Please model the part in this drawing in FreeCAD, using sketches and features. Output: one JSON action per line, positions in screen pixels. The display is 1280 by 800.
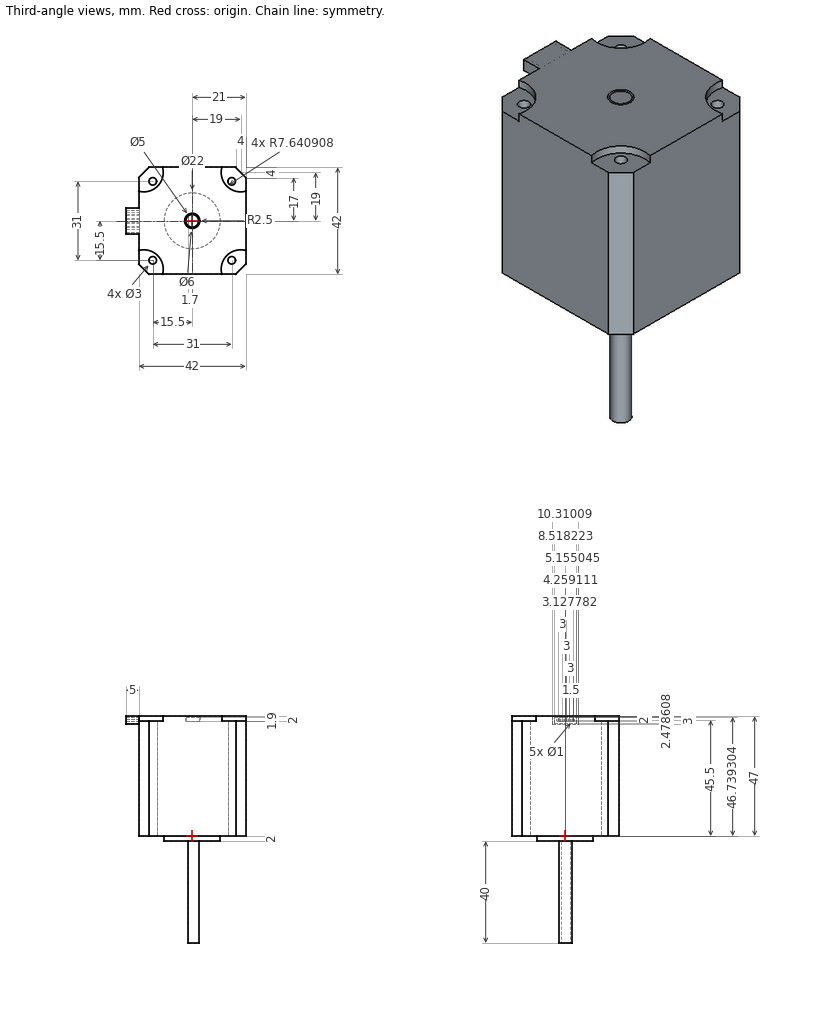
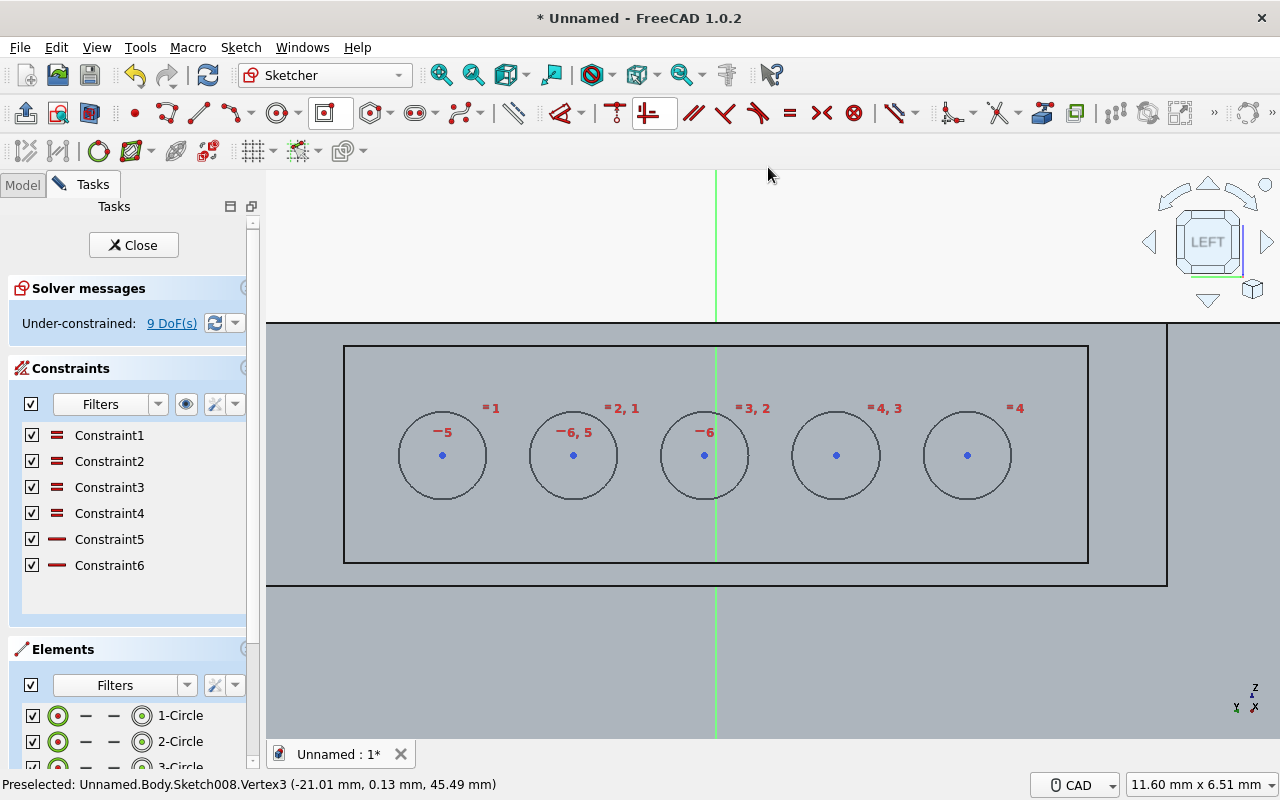
{"action": "left_click", "coordinate": [705, 456]}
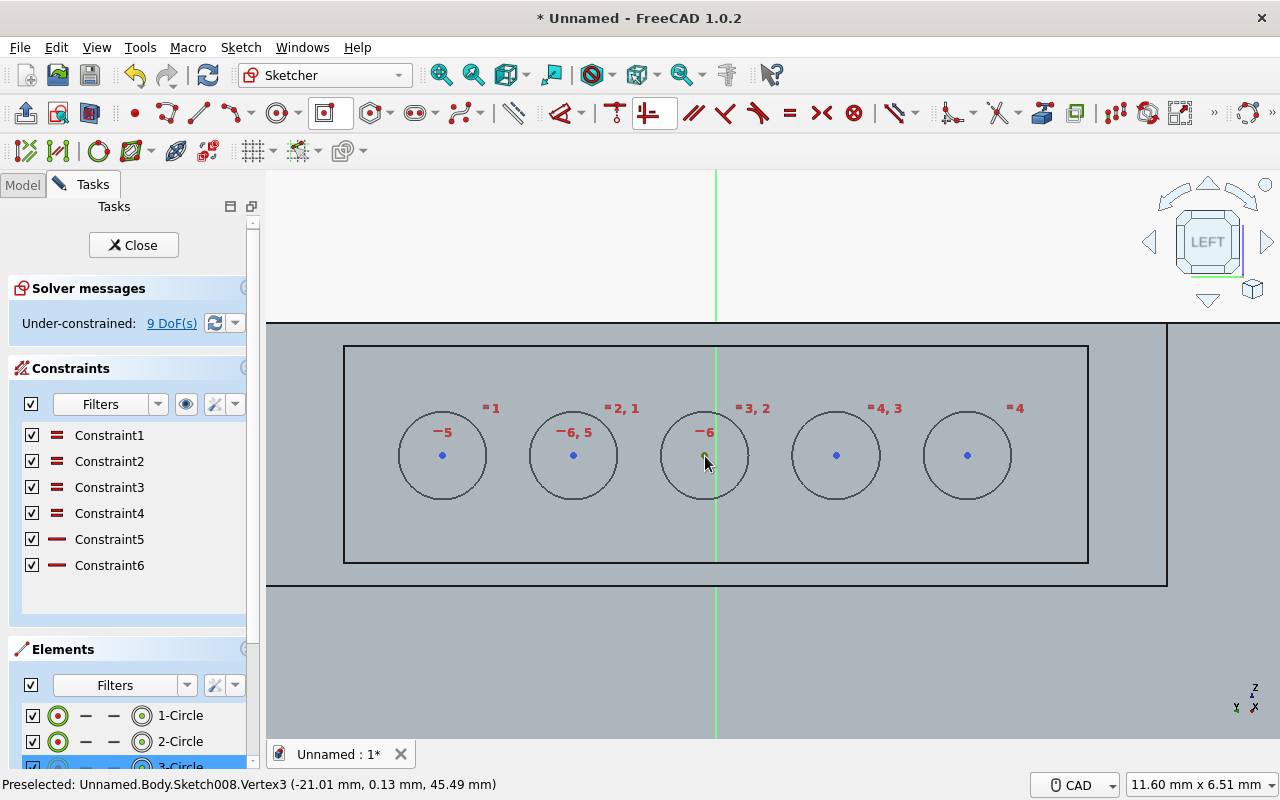
{"action": "left_click", "coordinate": [836, 455]}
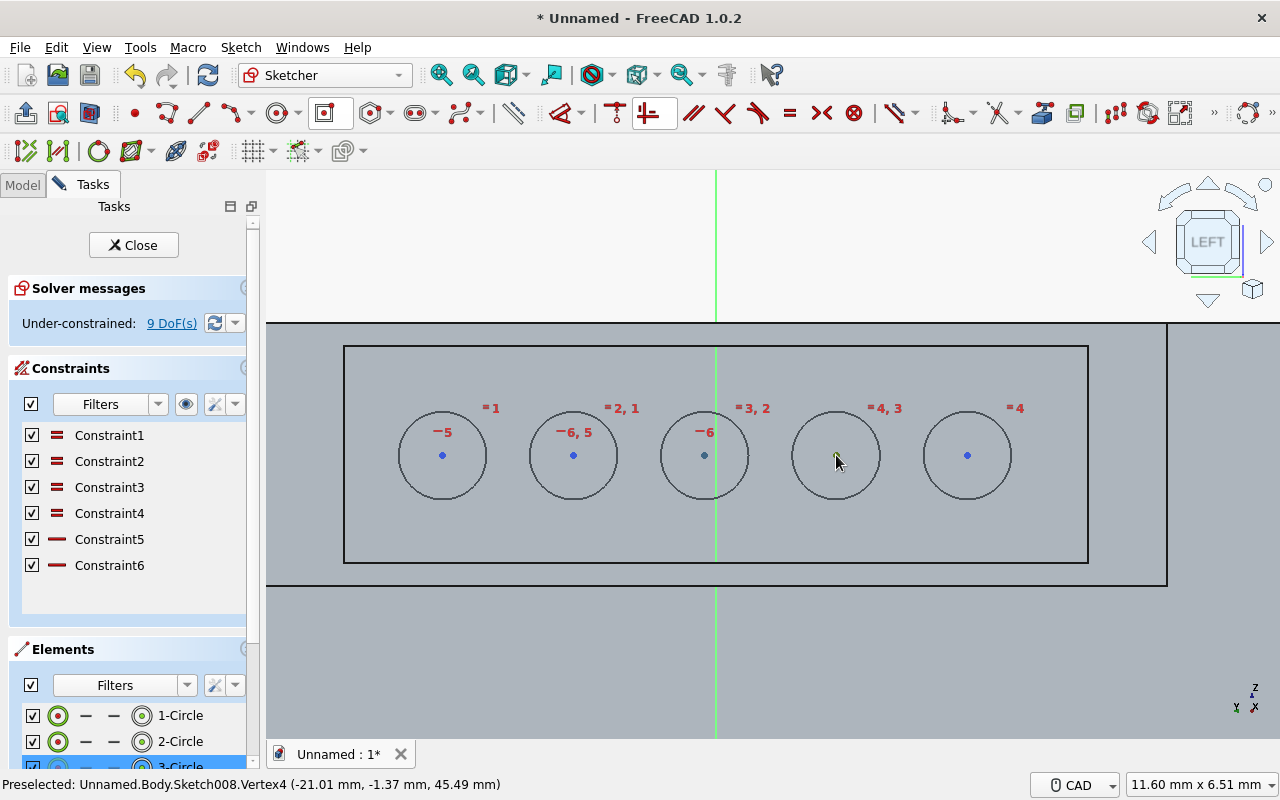
{"action": "key", "text": "h"}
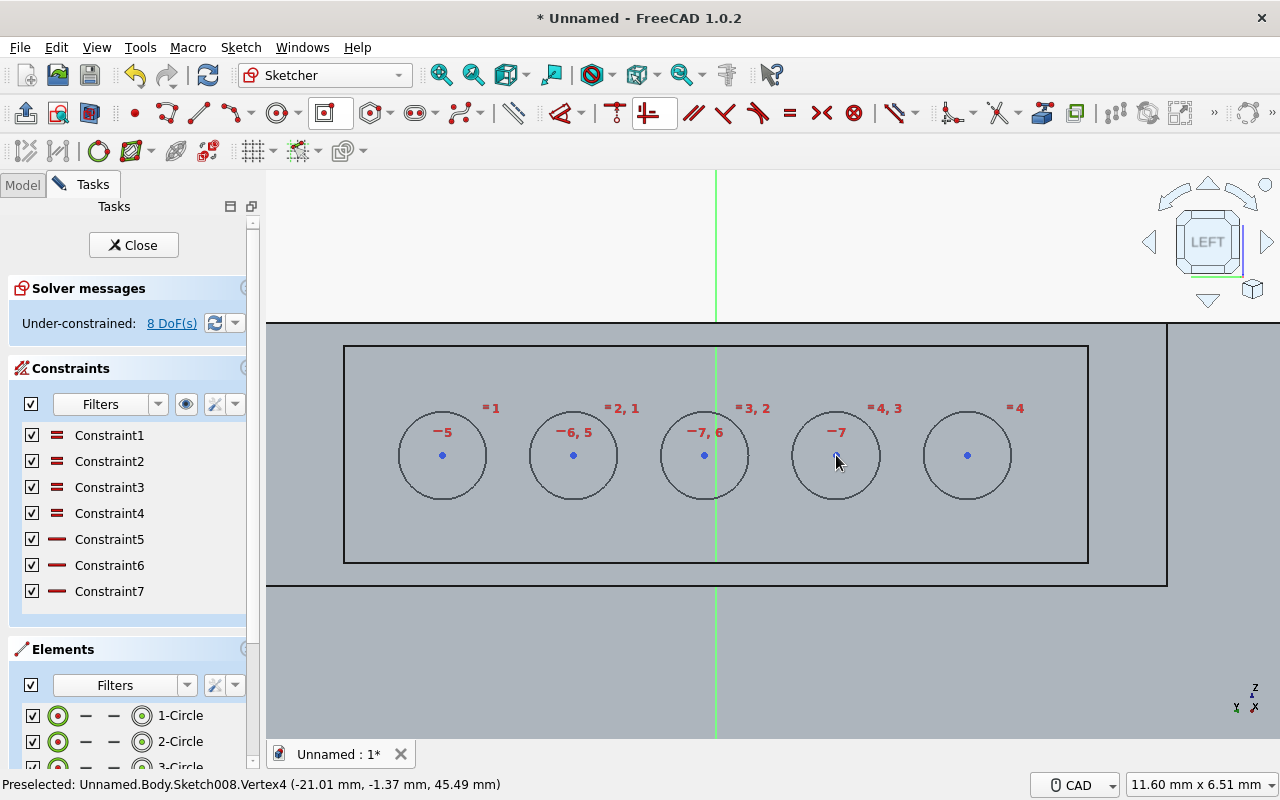
{"action": "left_click", "coordinate": [836, 456]}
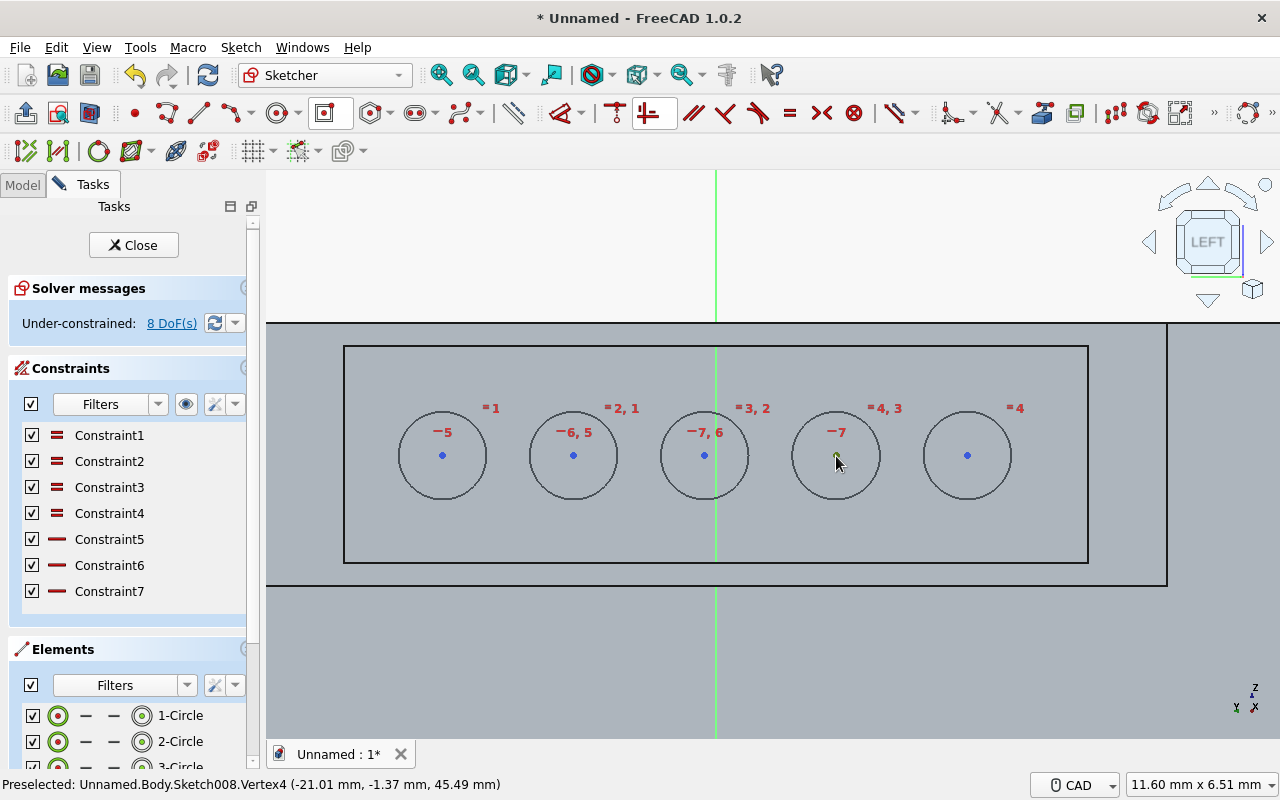
{"action": "left_click", "coordinate": [967, 455]}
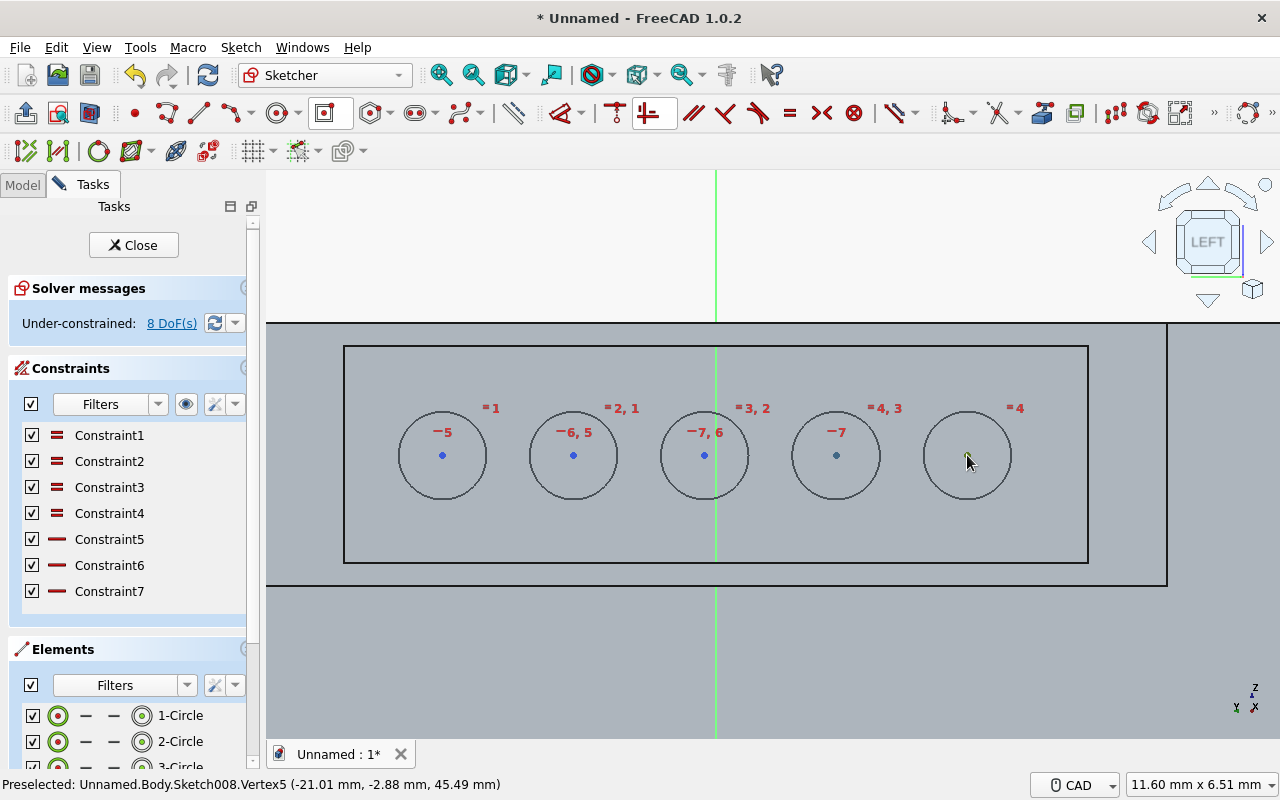
{"action": "left_click", "coordinate": [672, 114]}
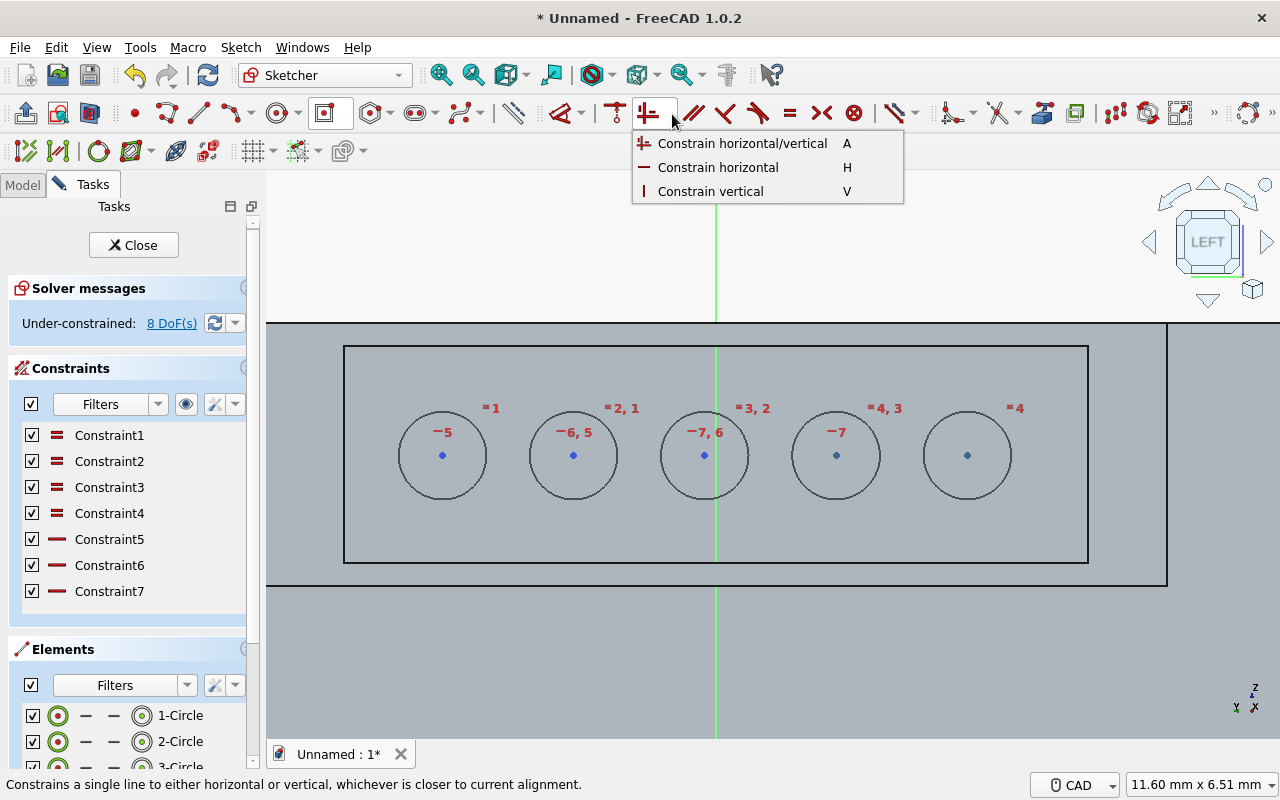
{"action": "left_click", "coordinate": [768, 167]}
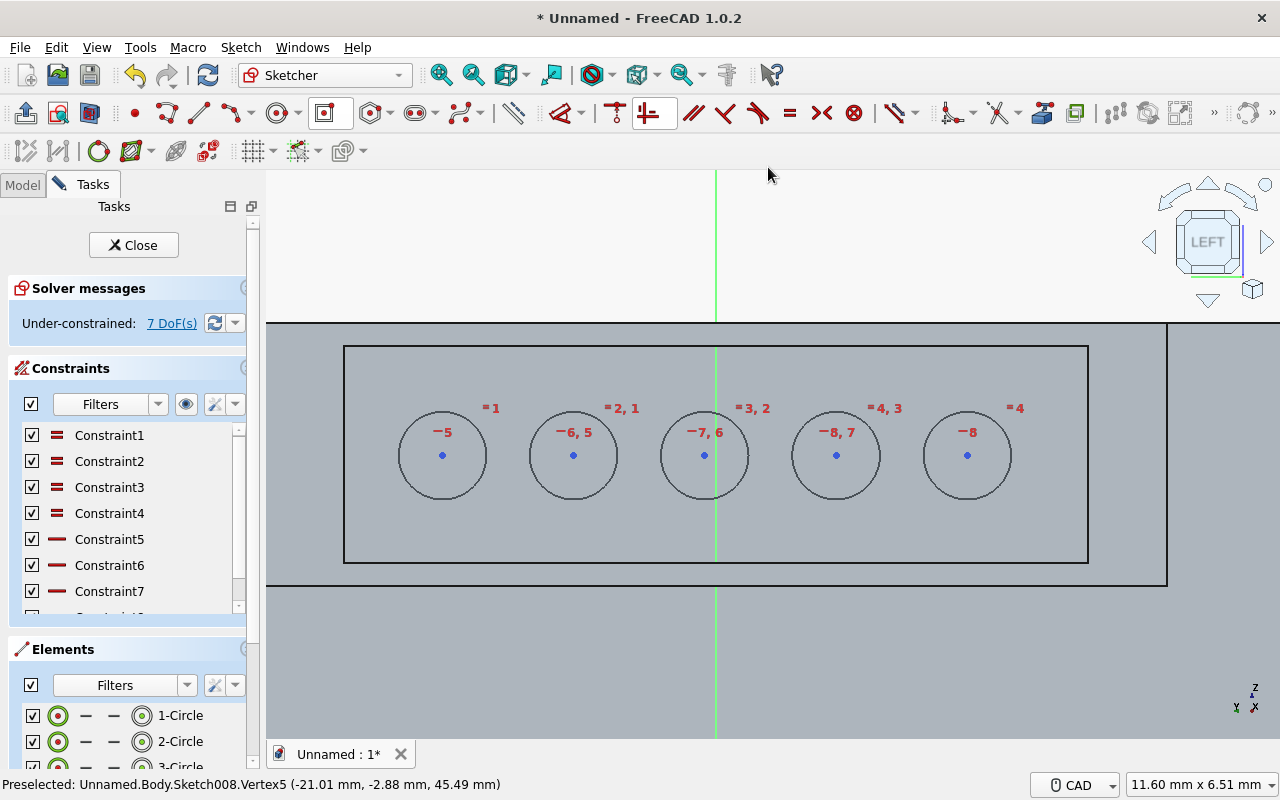
{"action": "left_click", "coordinate": [560, 114]}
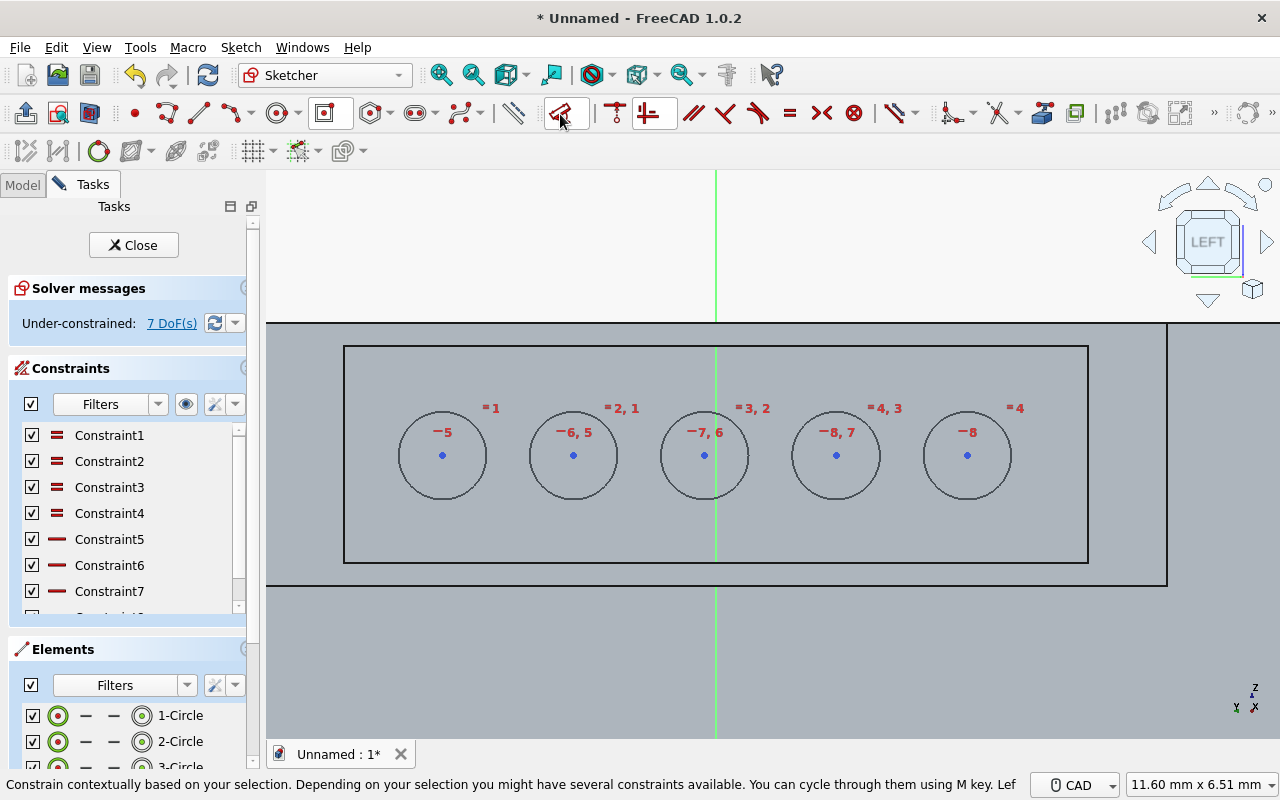
{"action": "left_click", "coordinate": [473, 425]}
{"action": "left_click", "coordinate": [496, 402]}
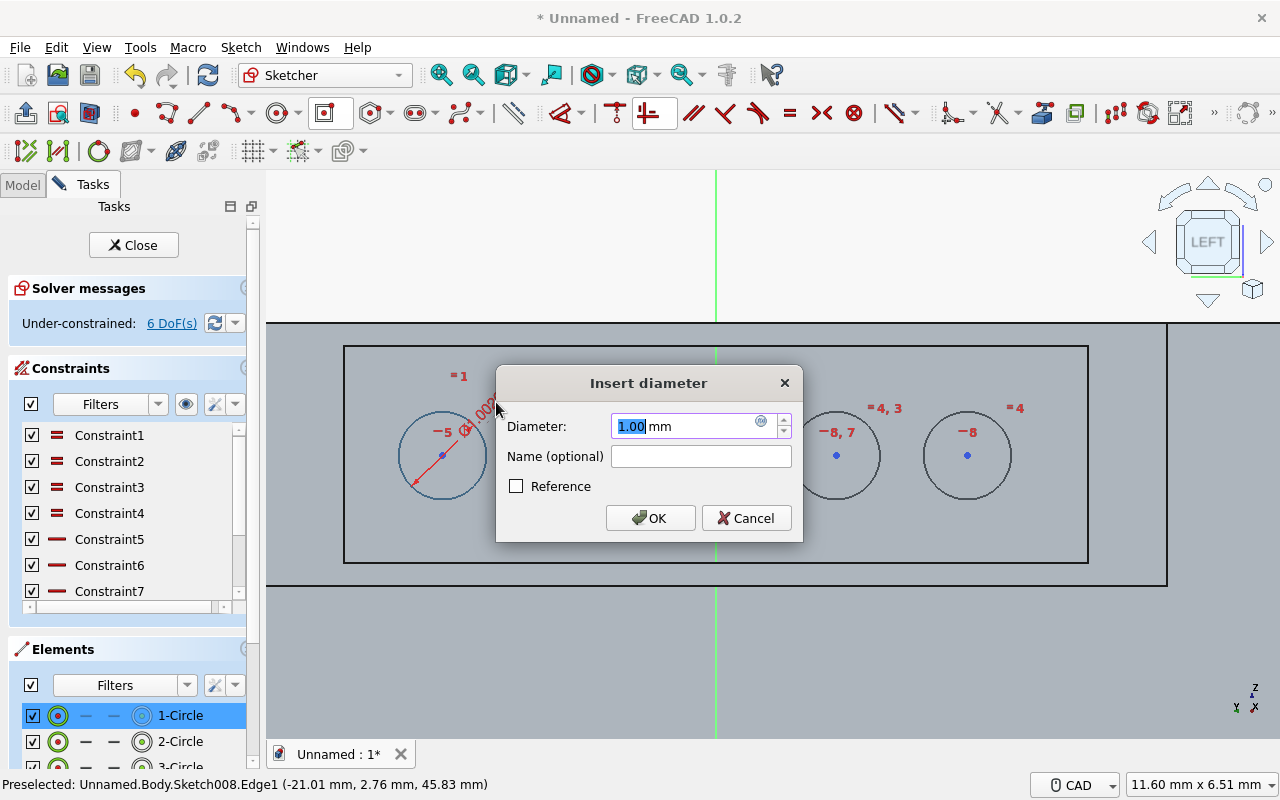
{"action": "type", "text": "1"}
{"action": "key", "text": "Return"}